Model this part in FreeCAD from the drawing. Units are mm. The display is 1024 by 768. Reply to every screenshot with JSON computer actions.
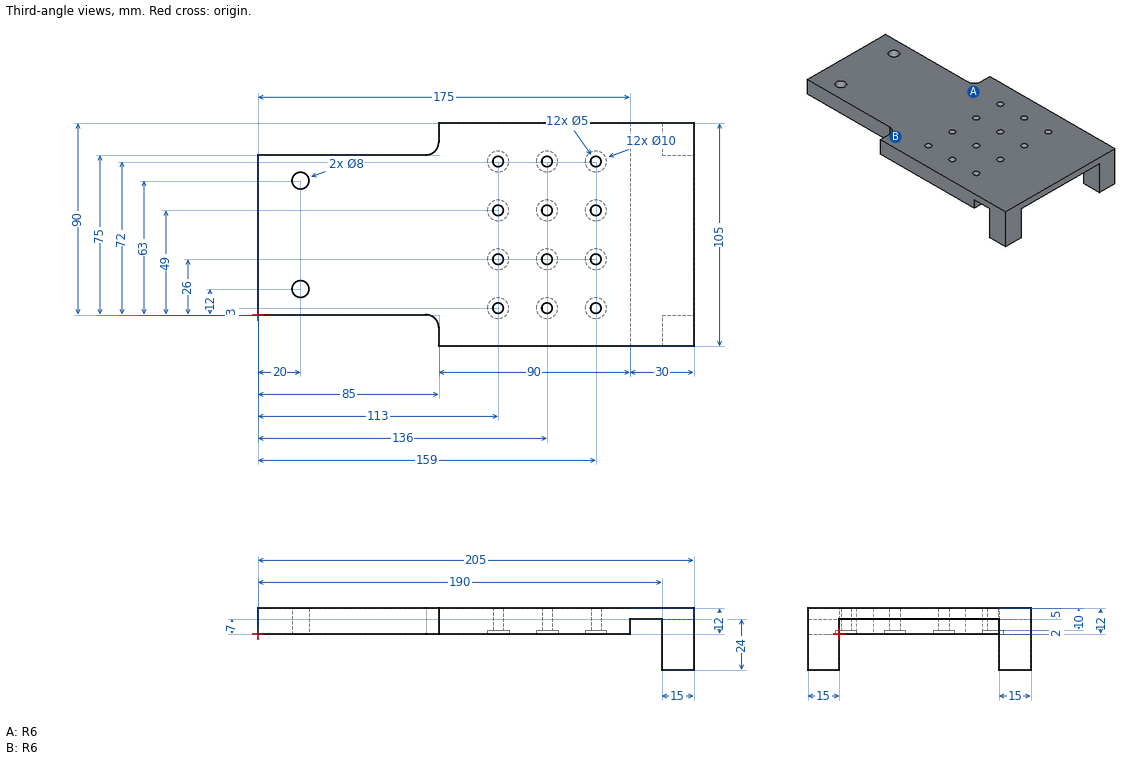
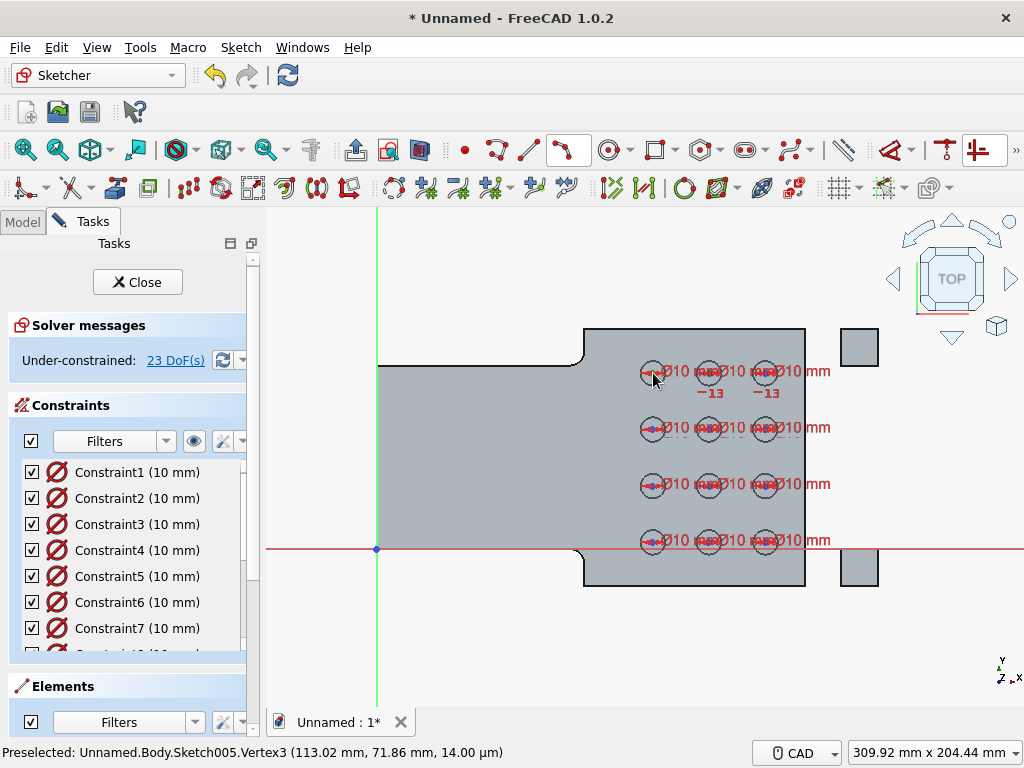
{"action": "key", "text": "h"}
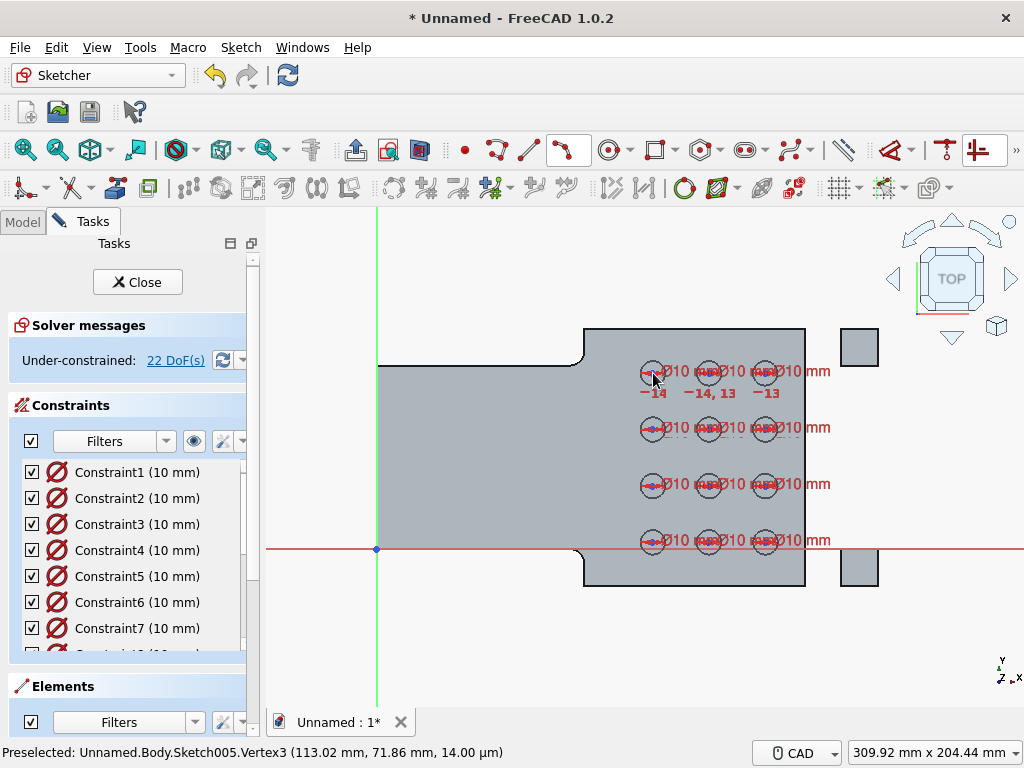
{"action": "left_click", "coordinate": [653, 373]}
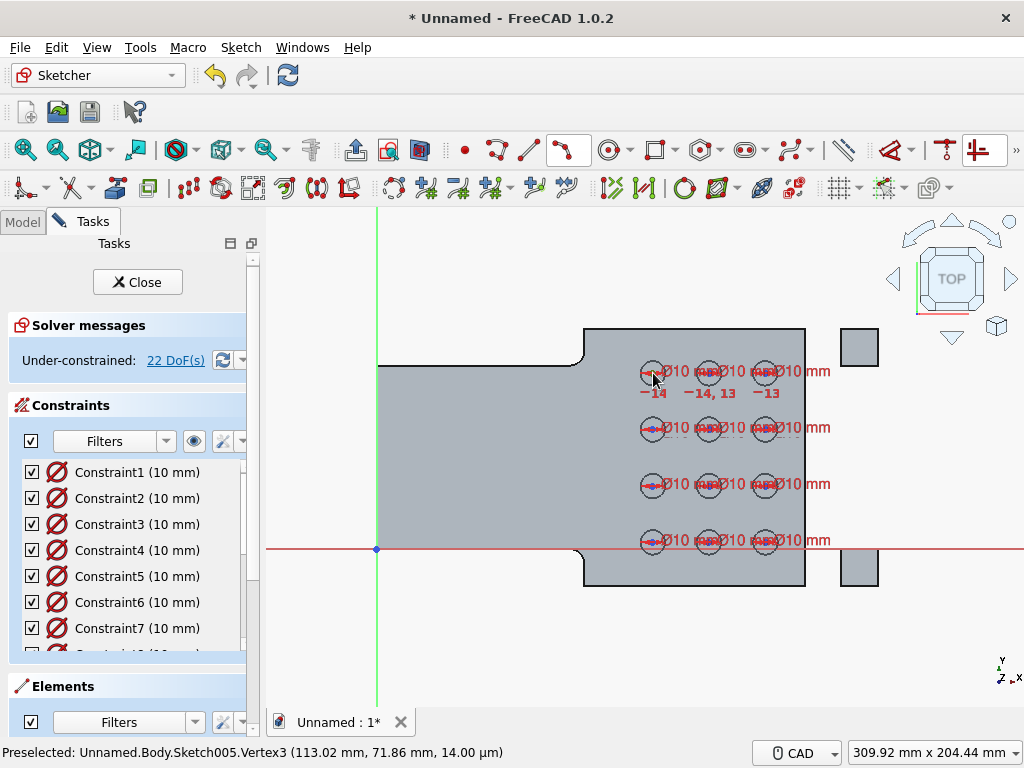
{"action": "left_click", "coordinate": [653, 430]}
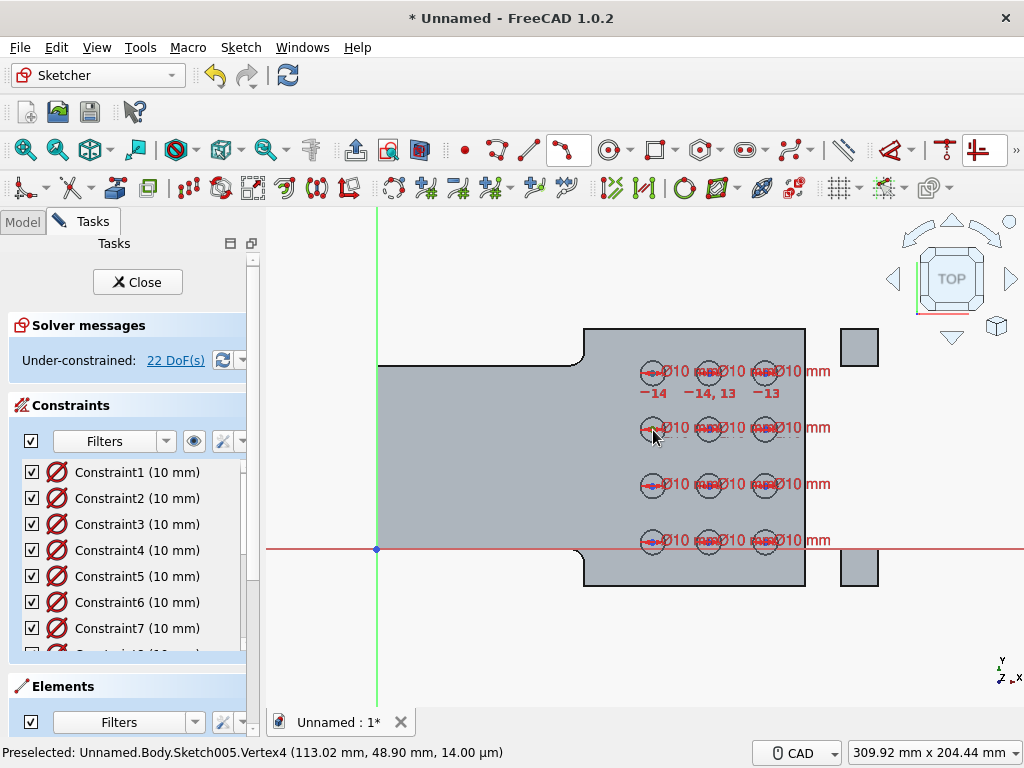
{"action": "key", "text": "v"}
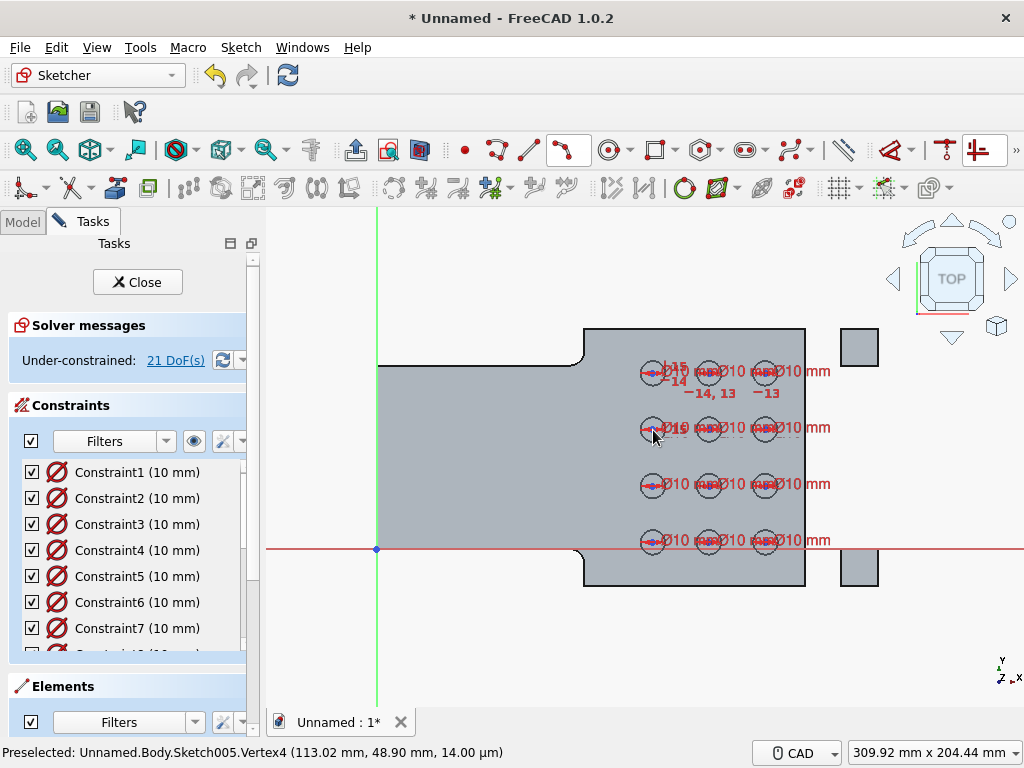
{"action": "left_click", "coordinate": [709, 373]}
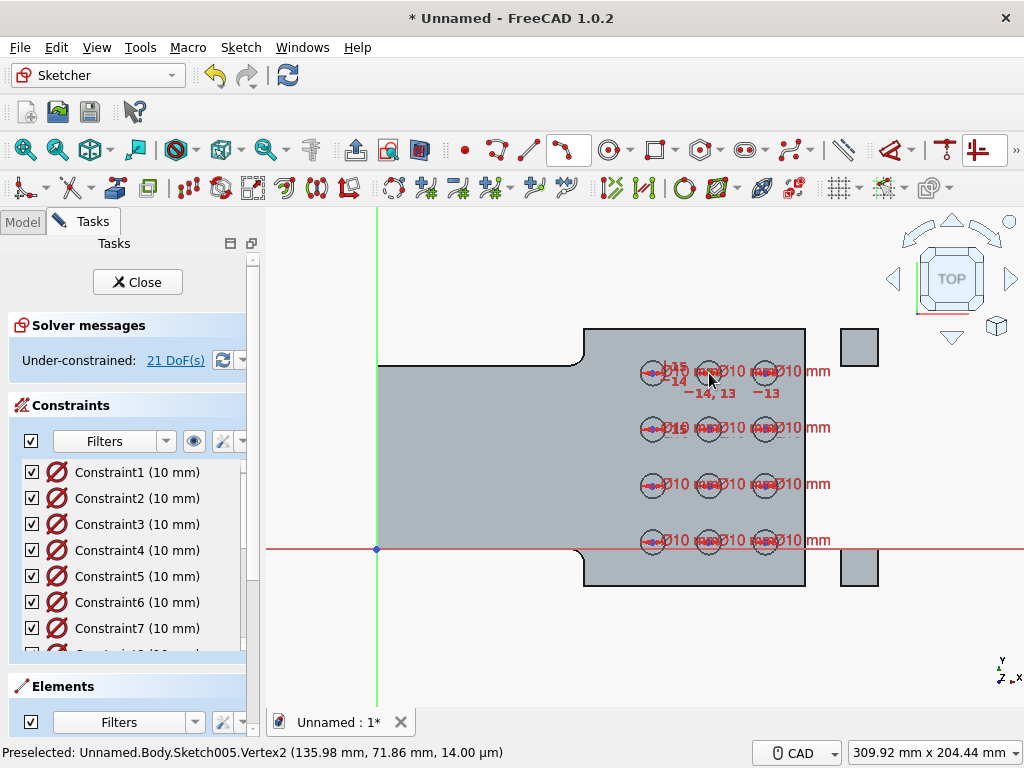
{"action": "left_click", "coordinate": [709, 430]}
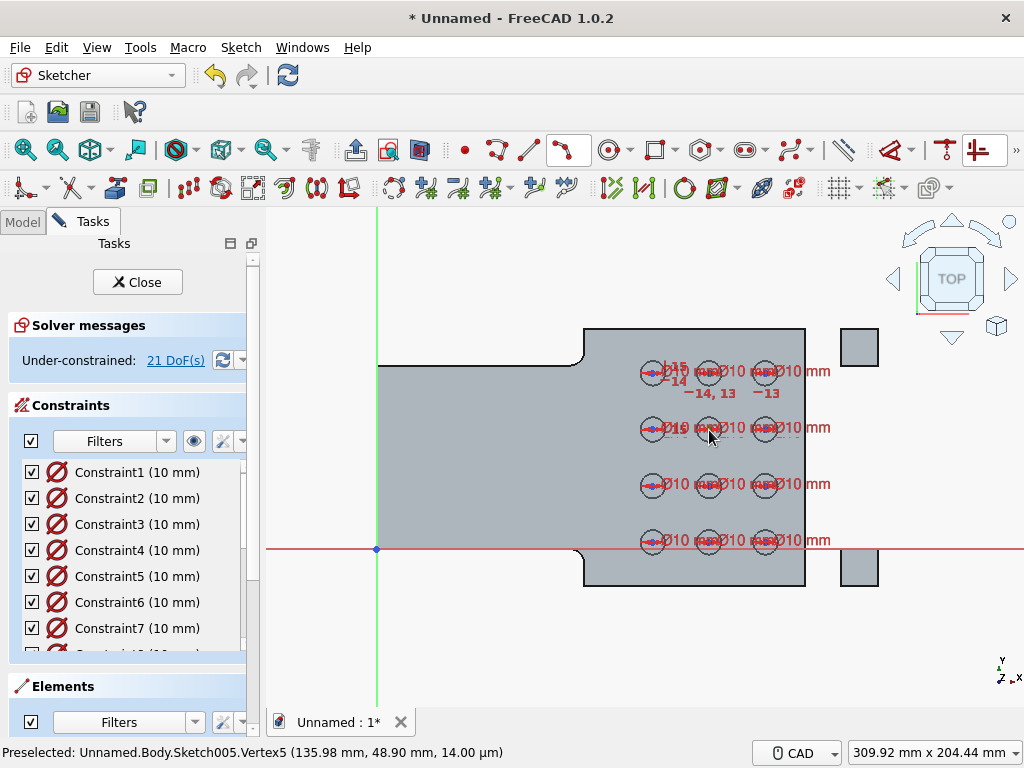
{"action": "key", "text": "v"}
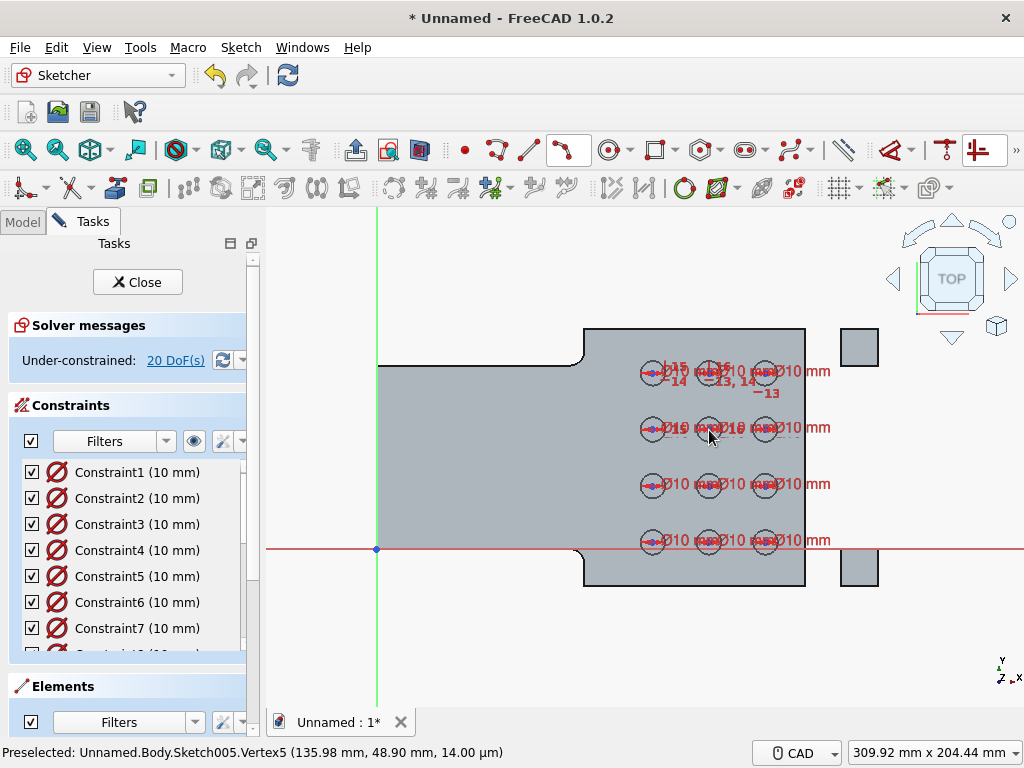
{"action": "left_click", "coordinate": [653, 430]}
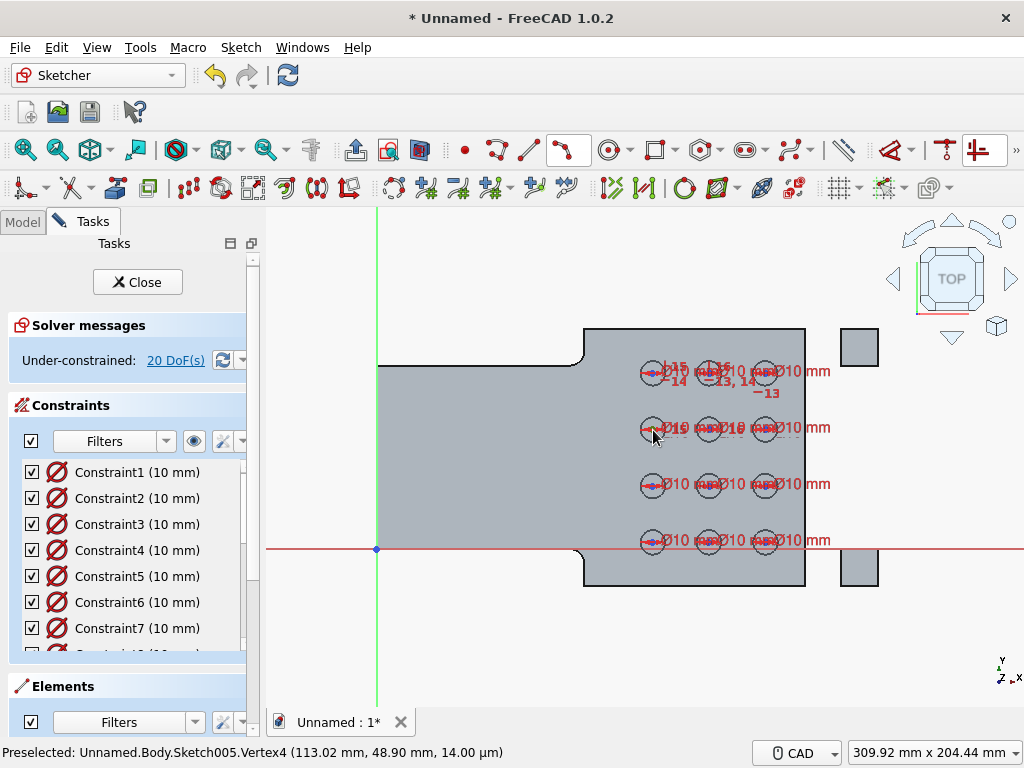
{"action": "left_click", "coordinate": [709, 430]}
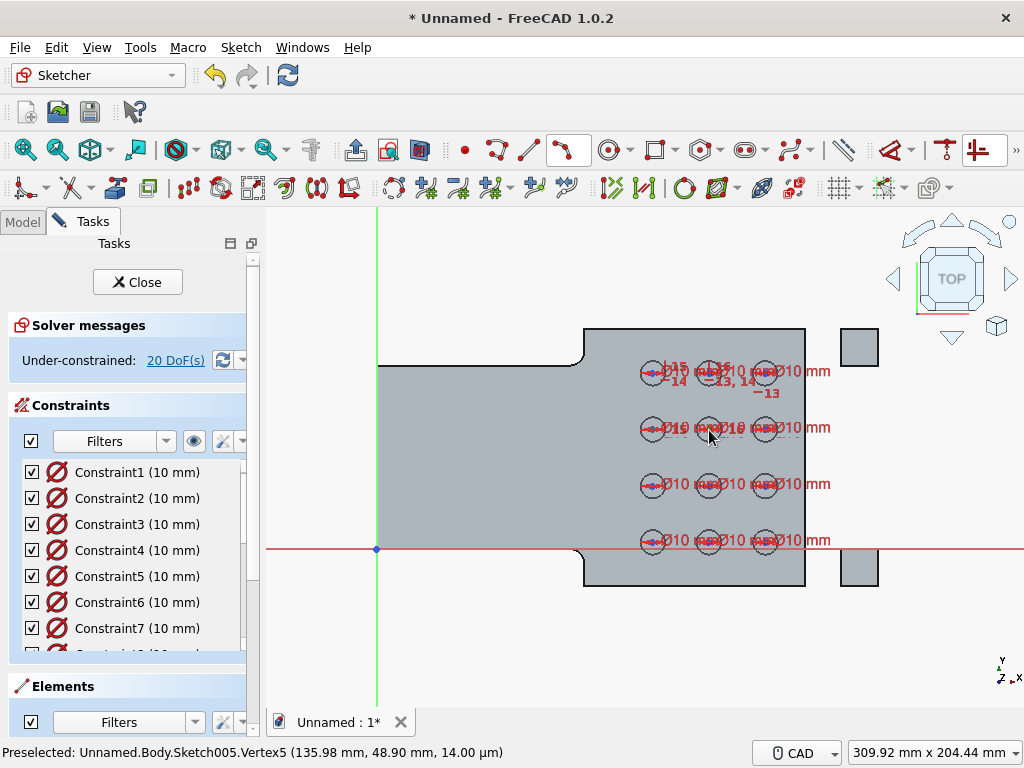
{"action": "left_click", "coordinate": [1002, 150]}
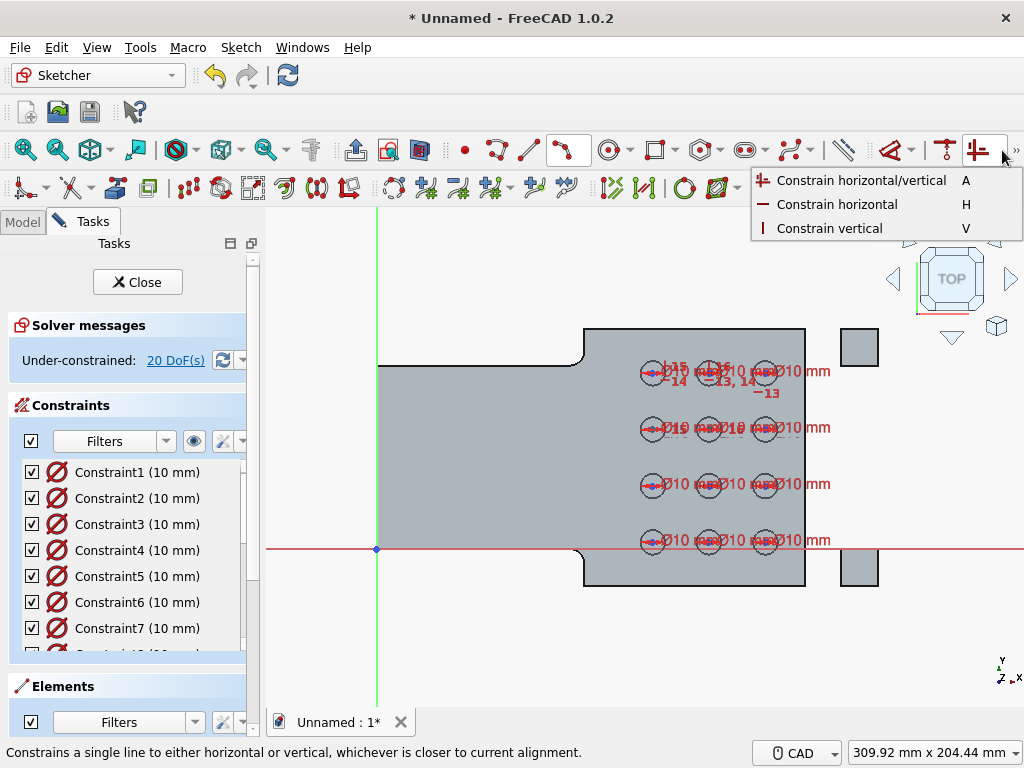
{"action": "left_click", "coordinate": [887, 204]}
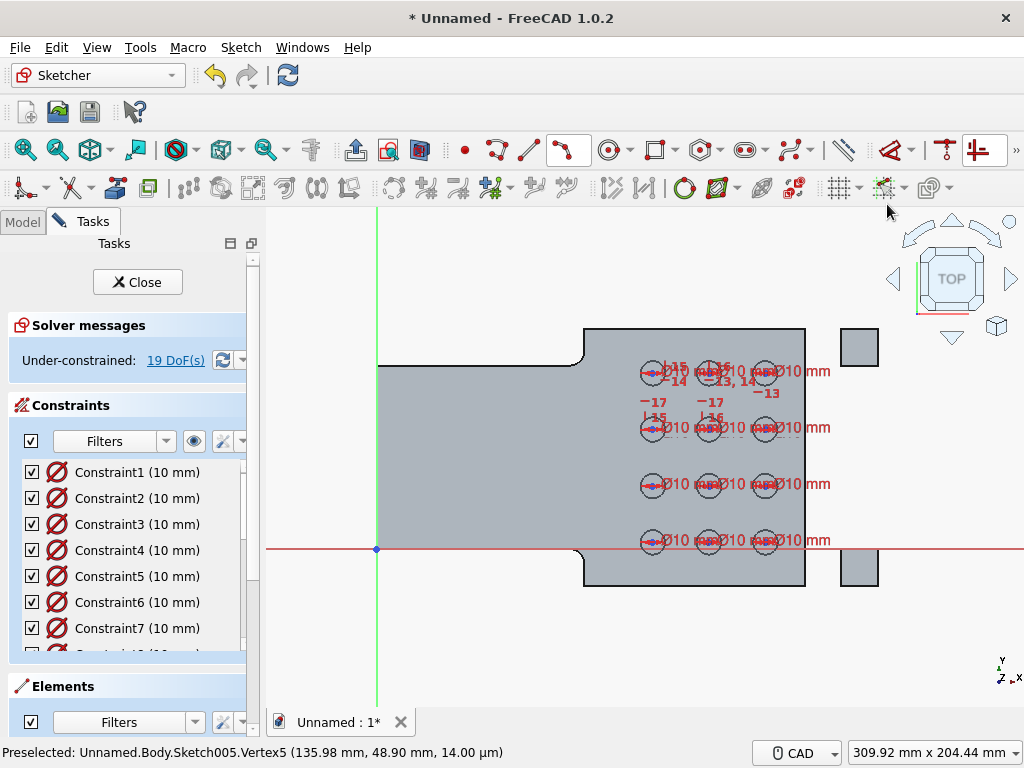
{"action": "left_click", "coordinate": [765, 373]}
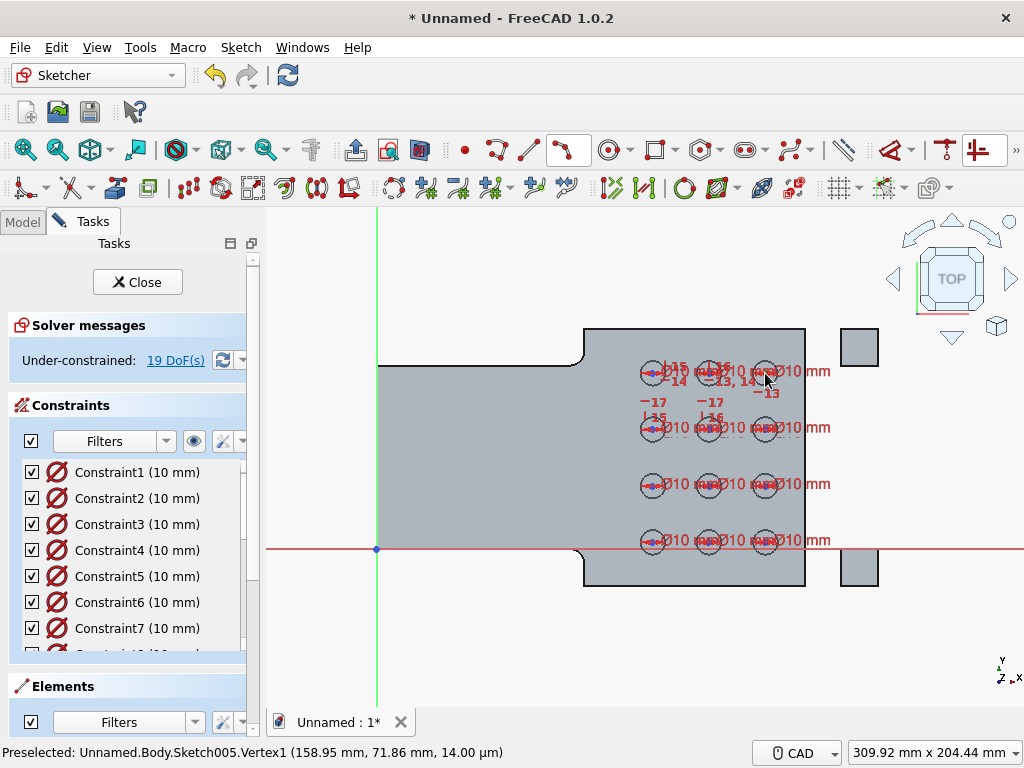
{"action": "left_click", "coordinate": [765, 430]}